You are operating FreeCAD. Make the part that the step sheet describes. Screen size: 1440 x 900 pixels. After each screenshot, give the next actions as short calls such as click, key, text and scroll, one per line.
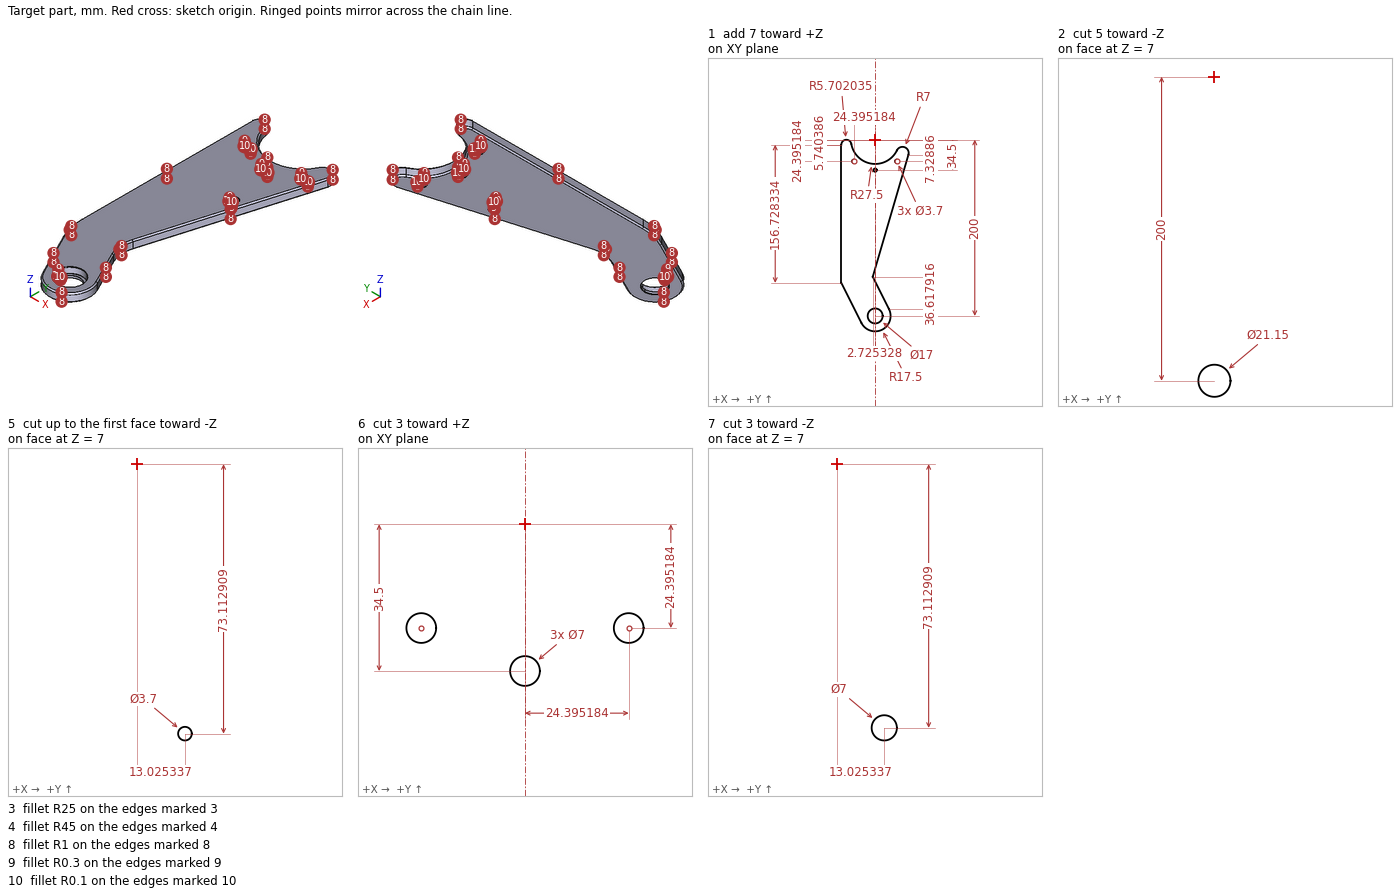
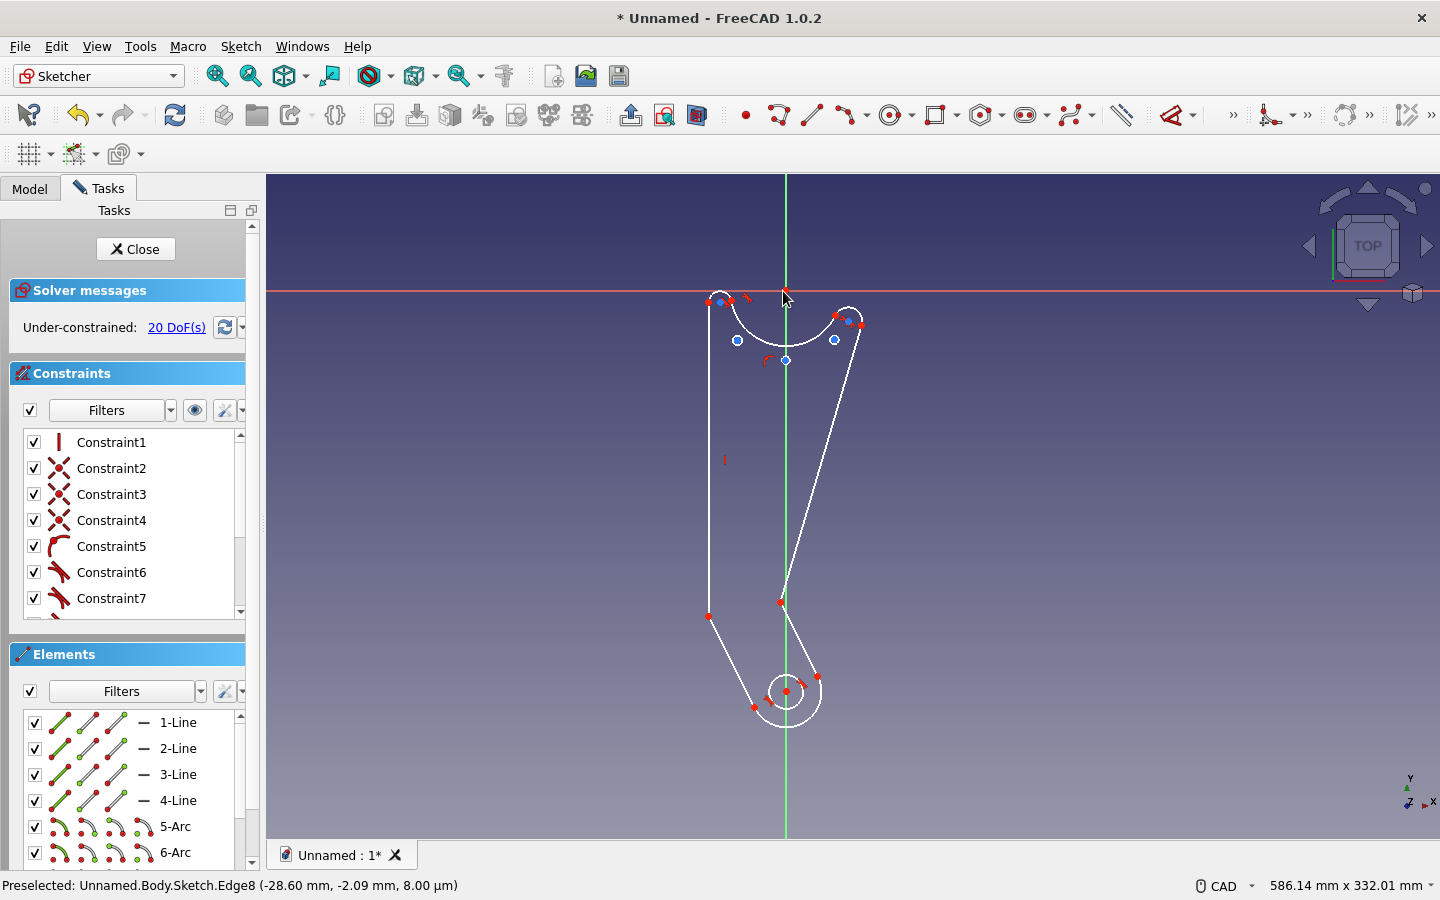
scroll(741, 337, up, 6)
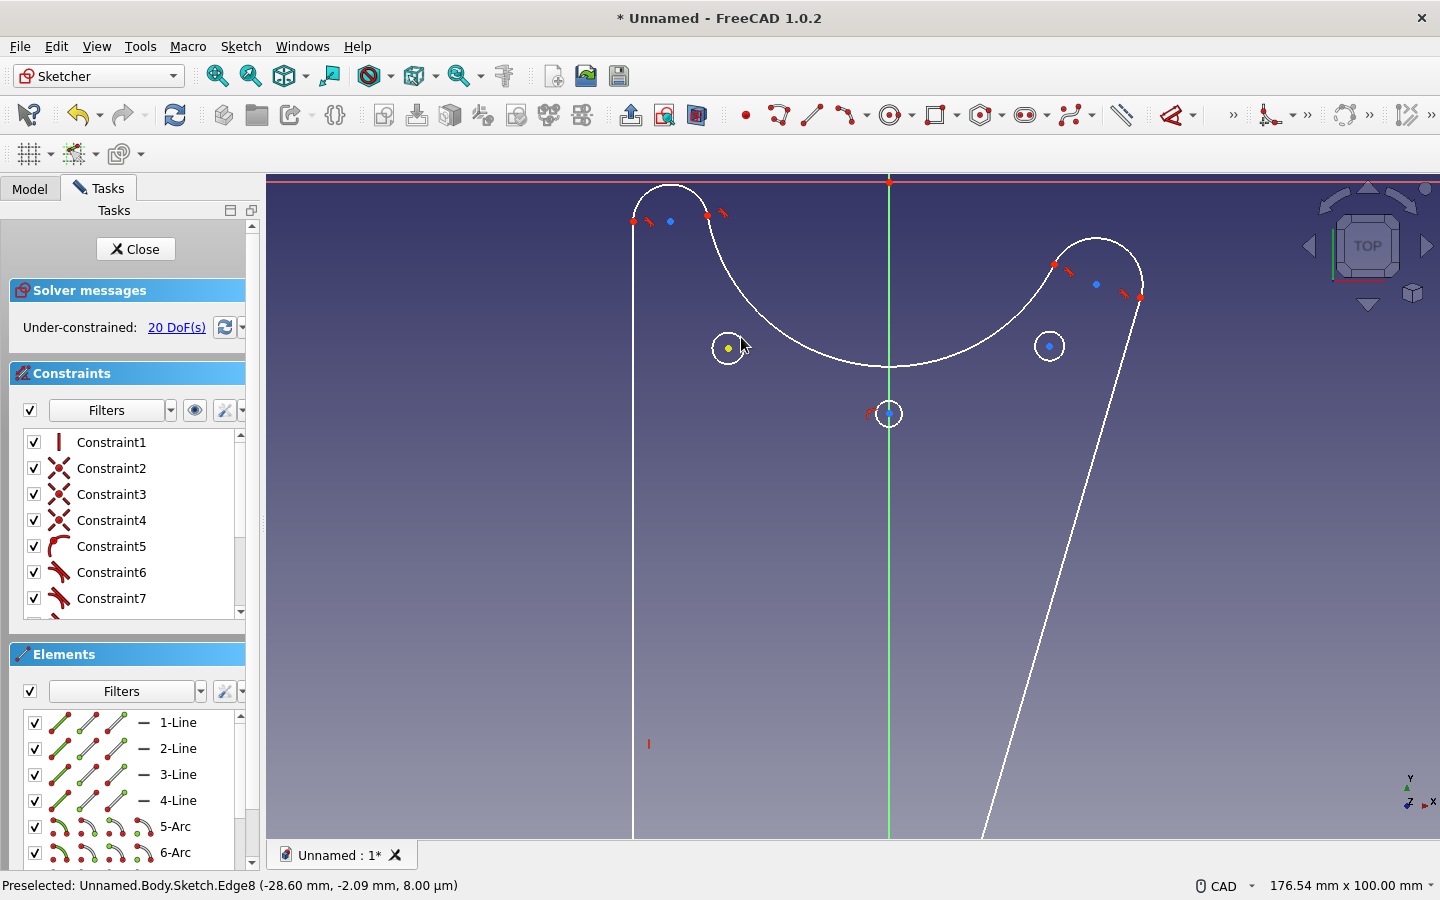
click(739, 337)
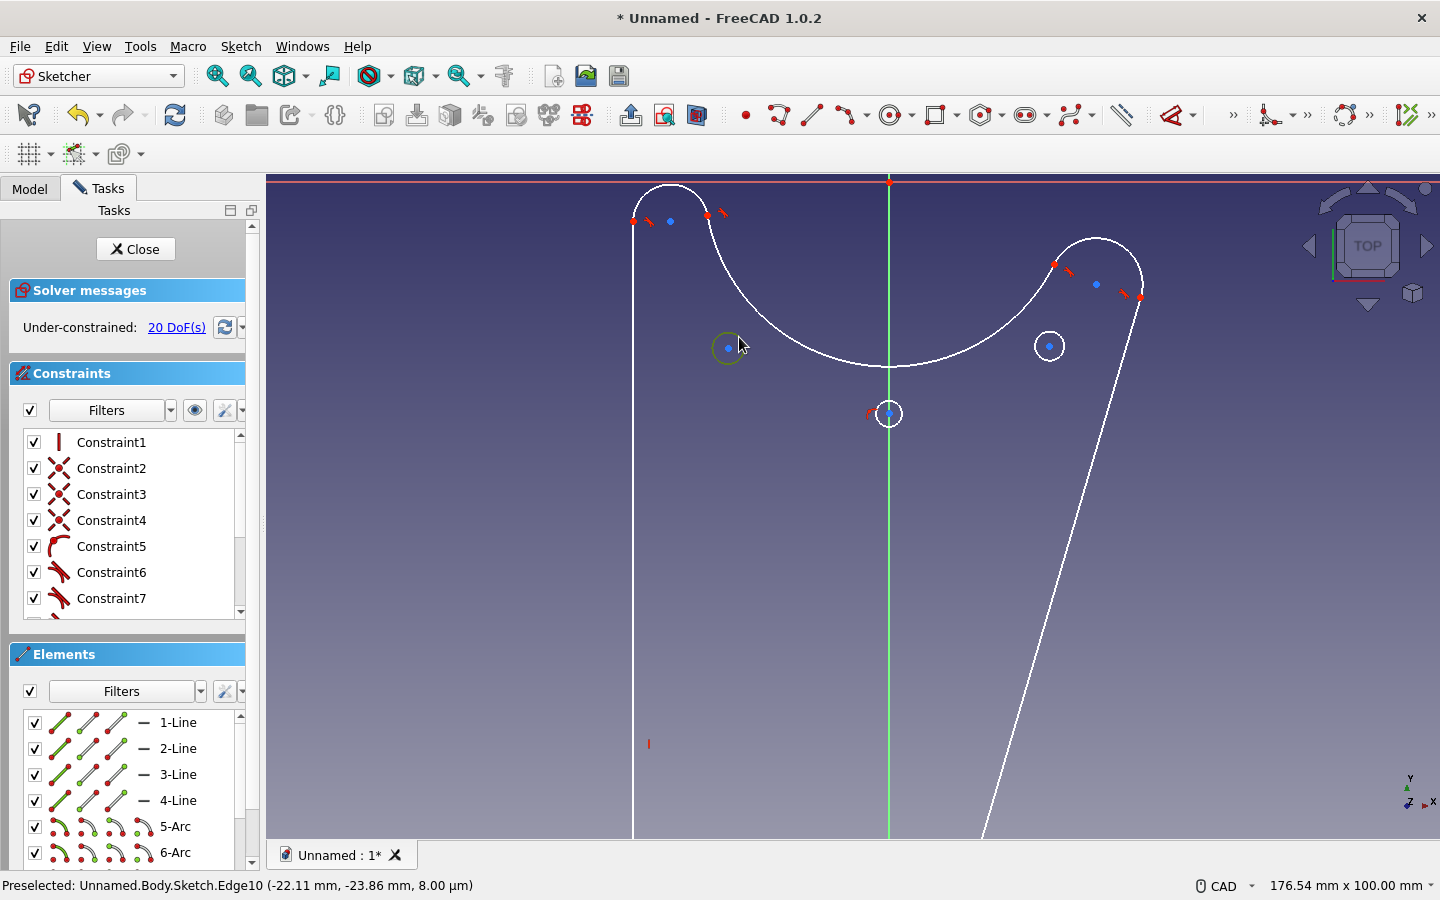
scroll(898, 405, up, 3)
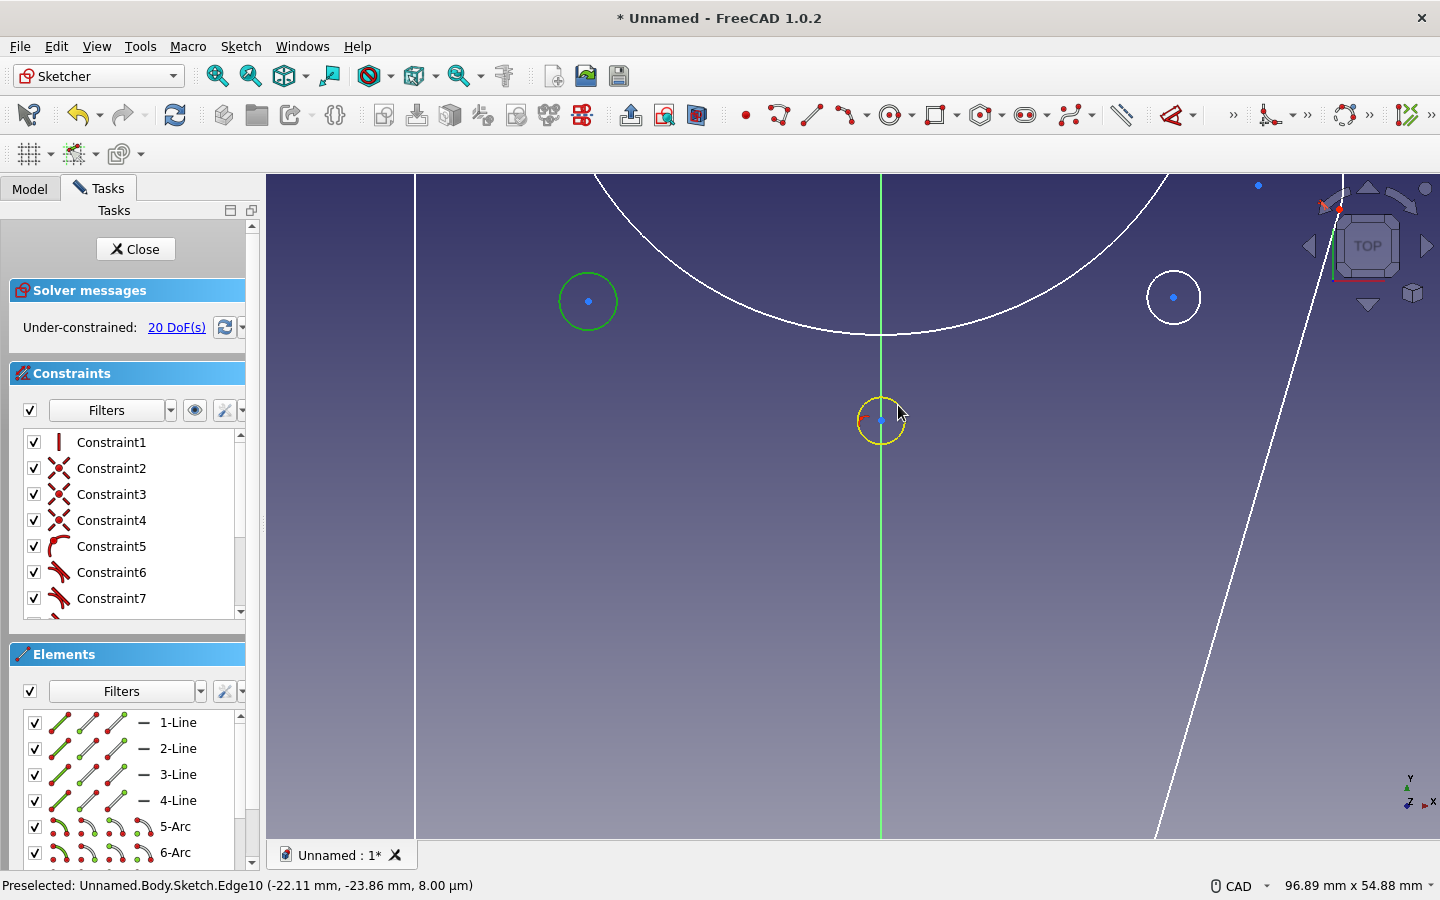
click(898, 404)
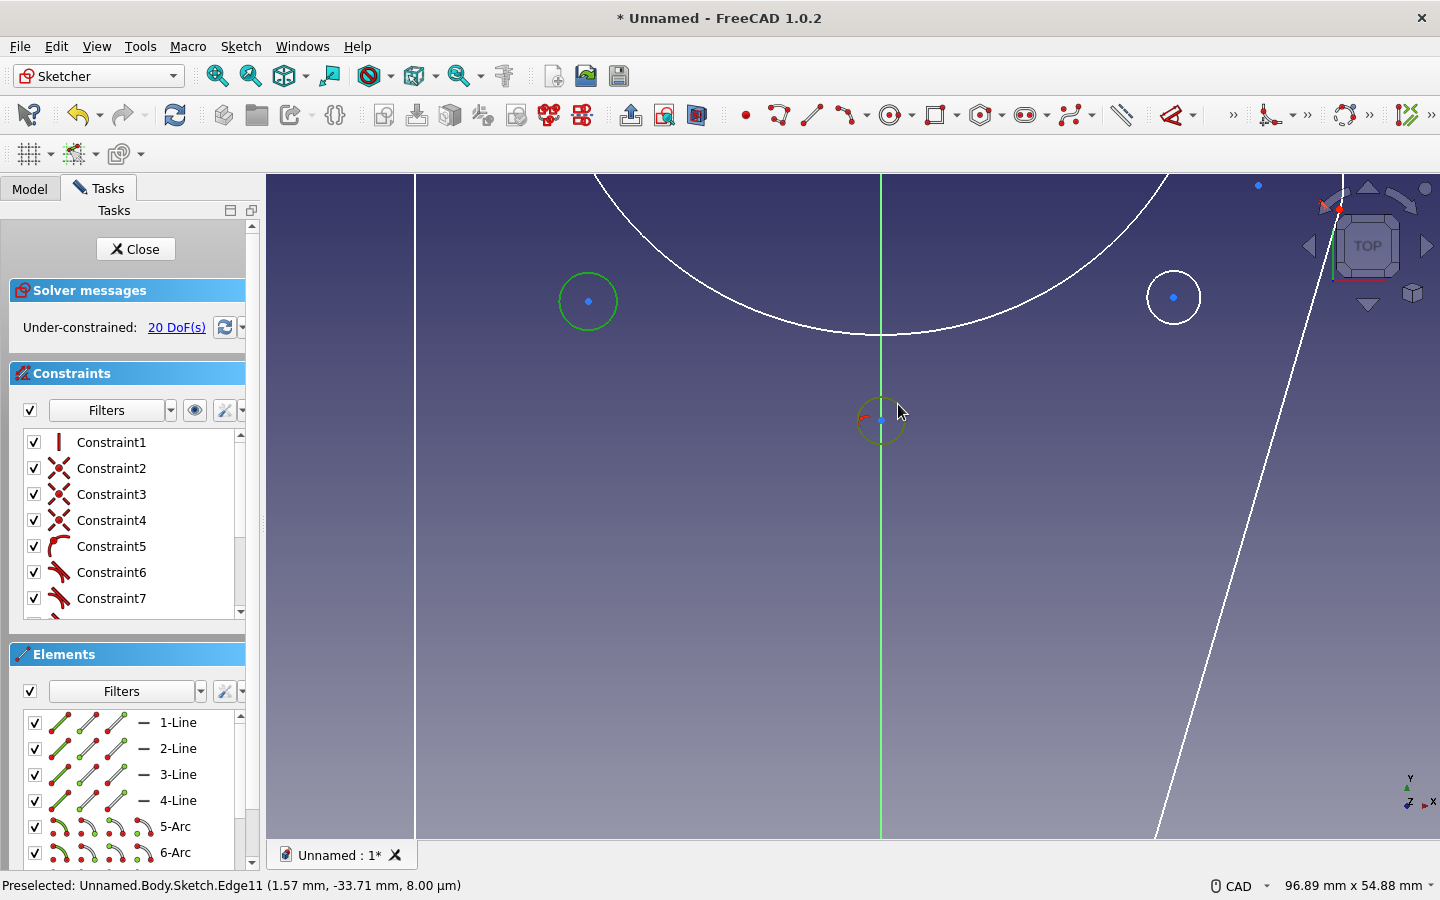
click(1193, 279)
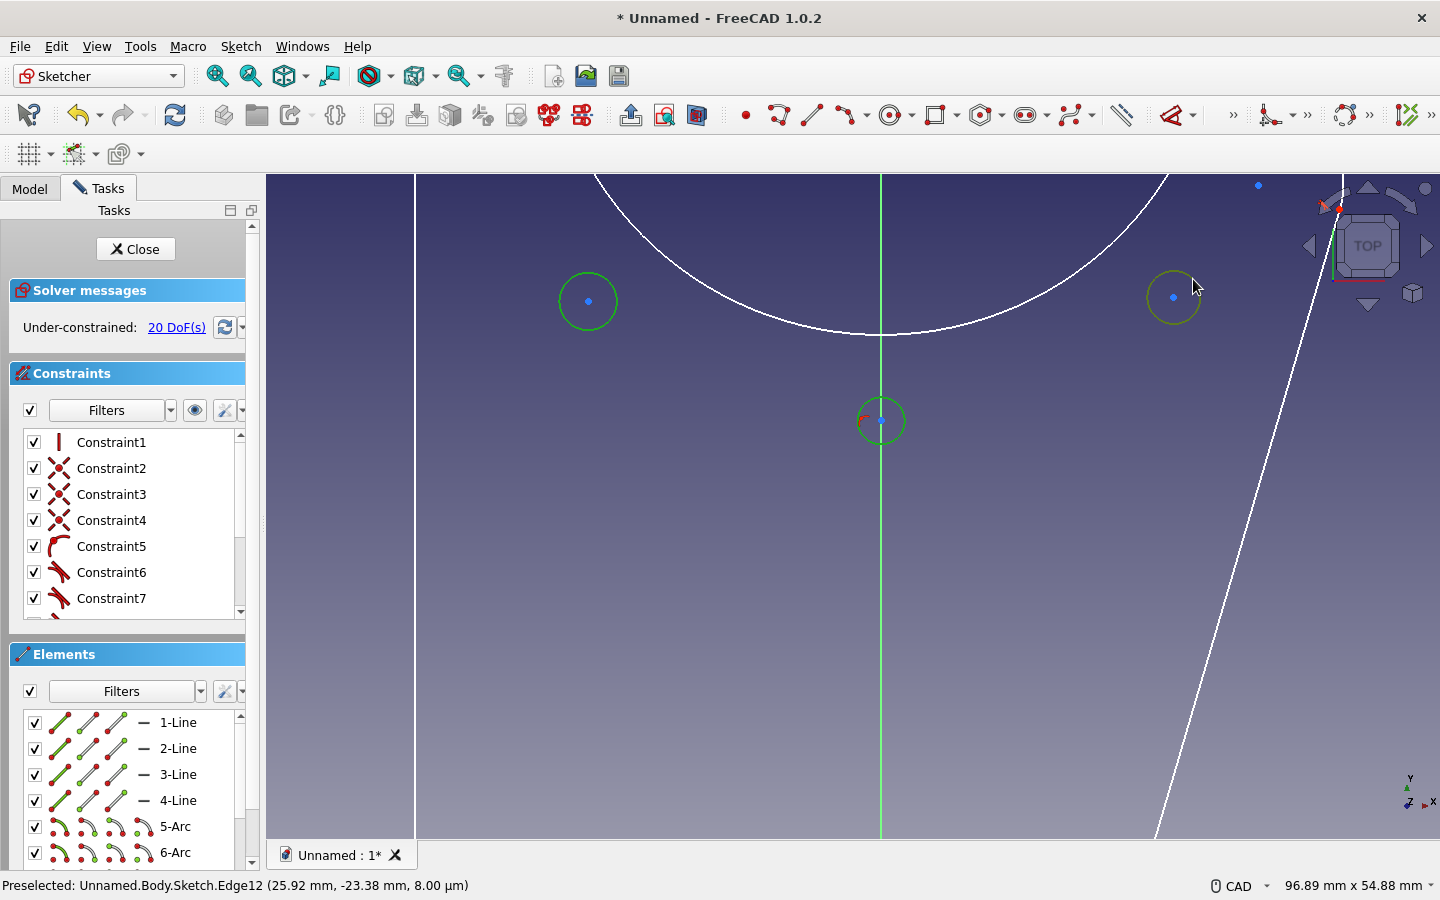
key(e)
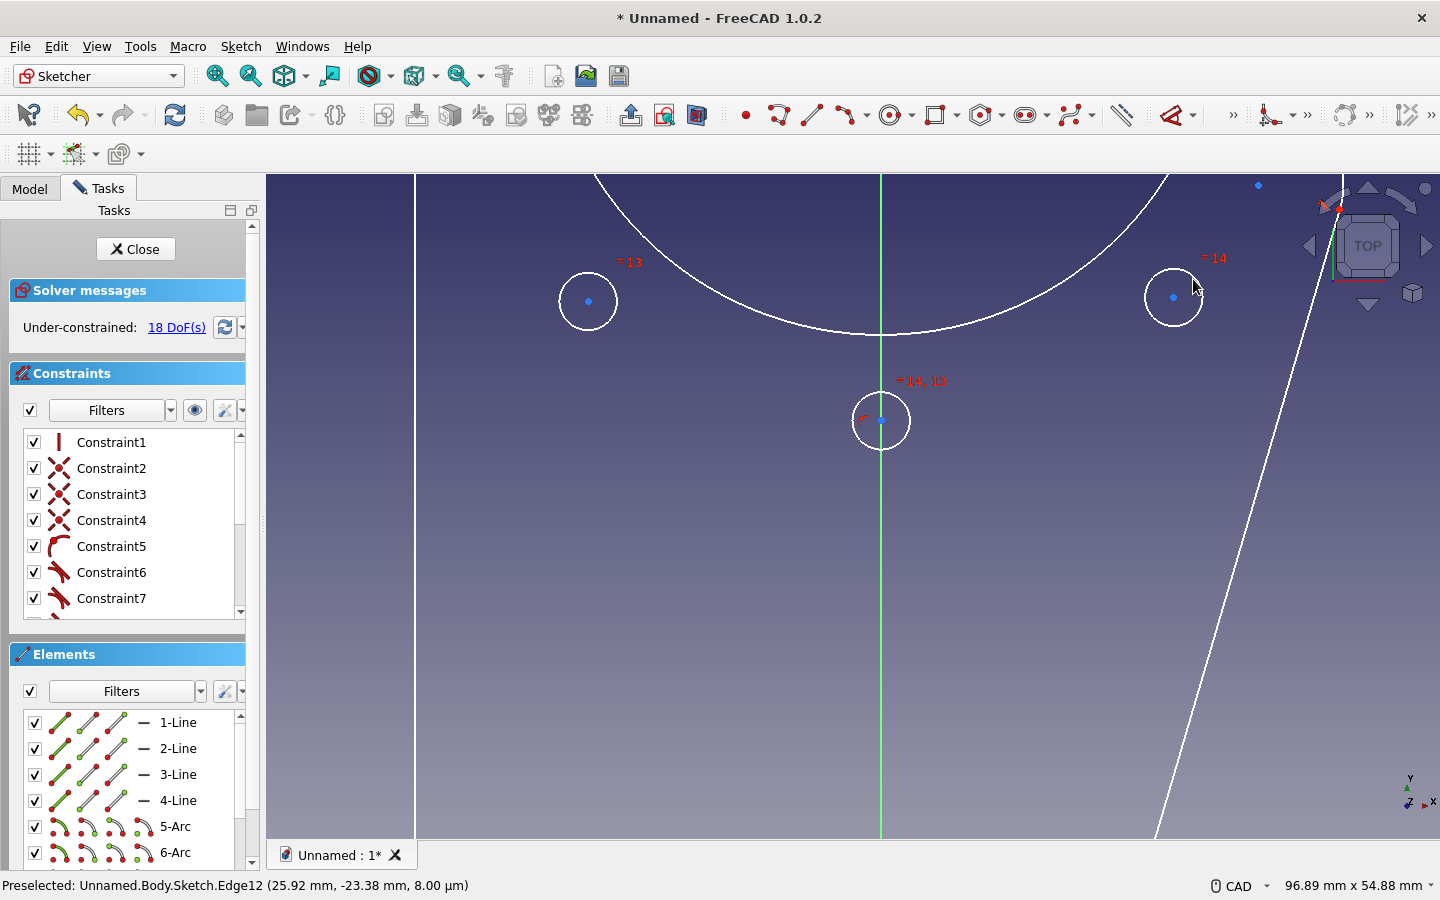
scroll(766, 348, down, 9)